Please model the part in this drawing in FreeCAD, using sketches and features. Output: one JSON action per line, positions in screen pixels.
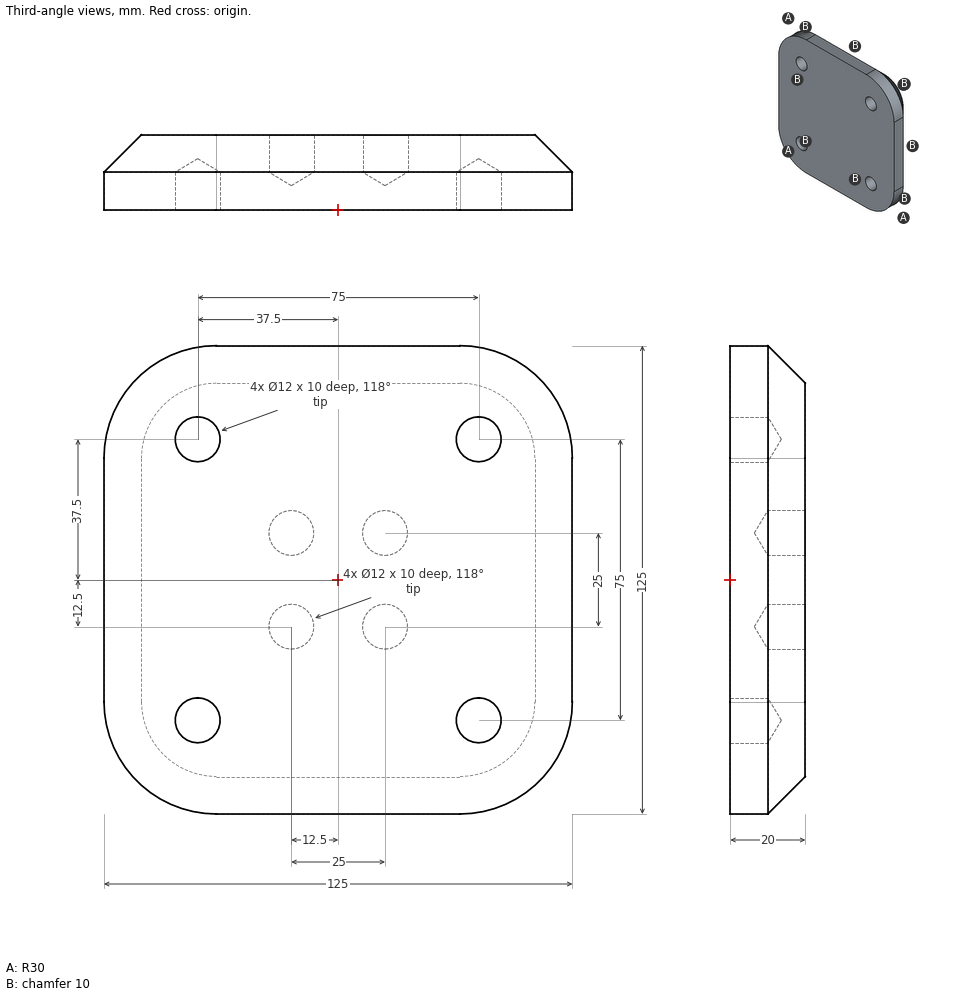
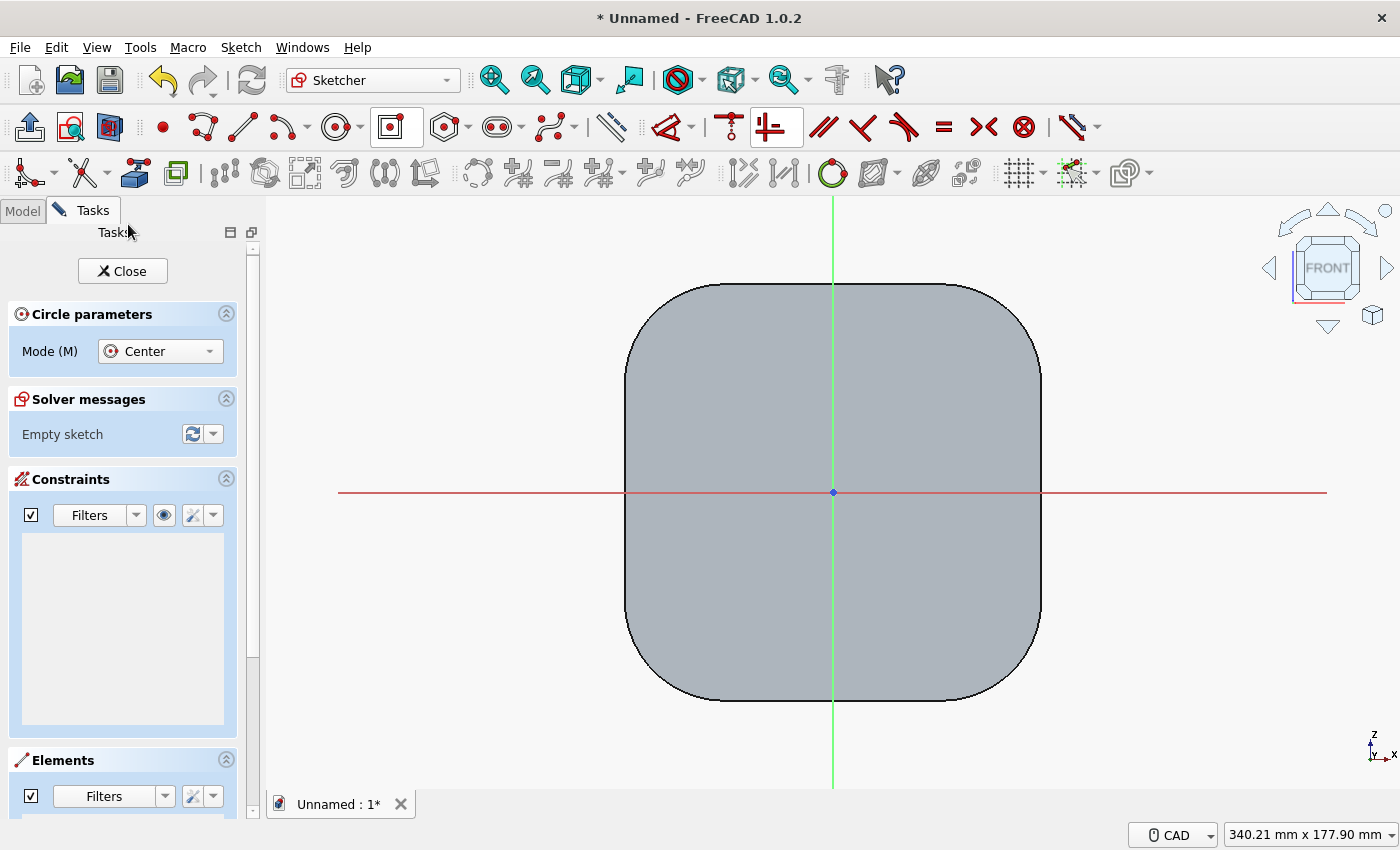
{"action": "left_click", "coordinate": [708, 368]}
{"action": "left_click", "coordinate": [722, 353]}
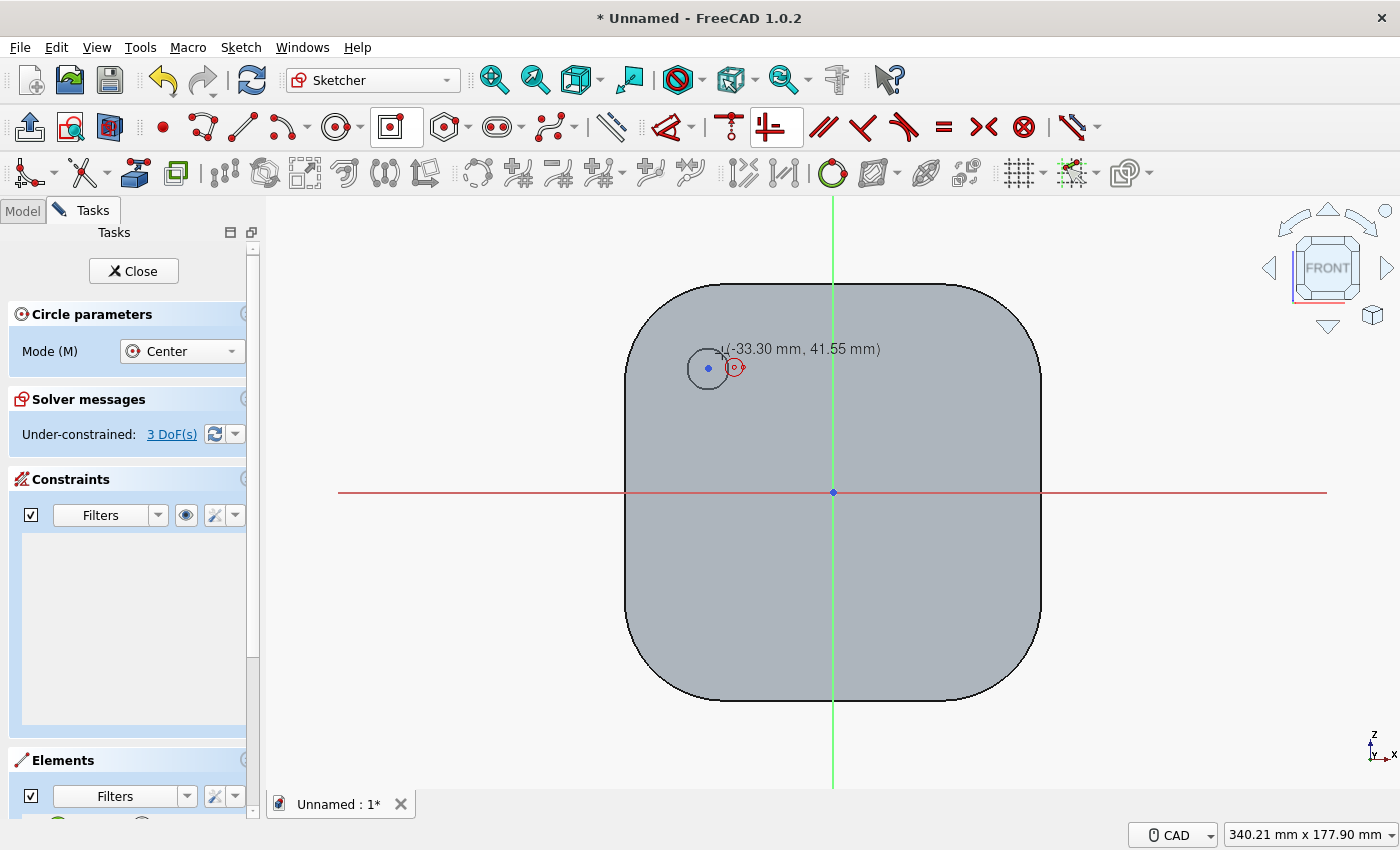
{"action": "left_click", "coordinate": [958, 368]}
{"action": "left_click", "coordinate": [972, 353]}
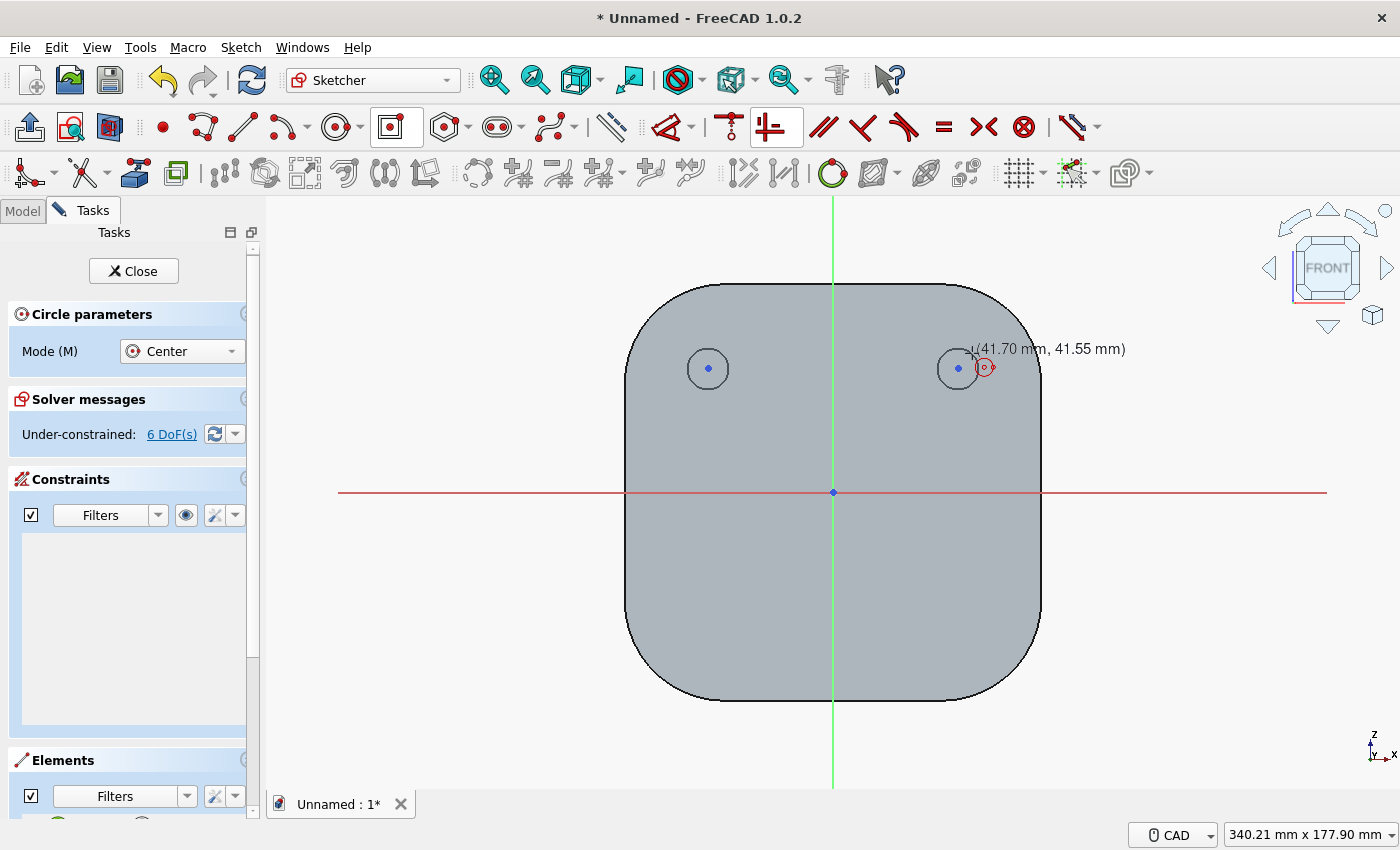
{"action": "left_click", "coordinate": [958, 617]}
{"action": "left_click", "coordinate": [972, 603]}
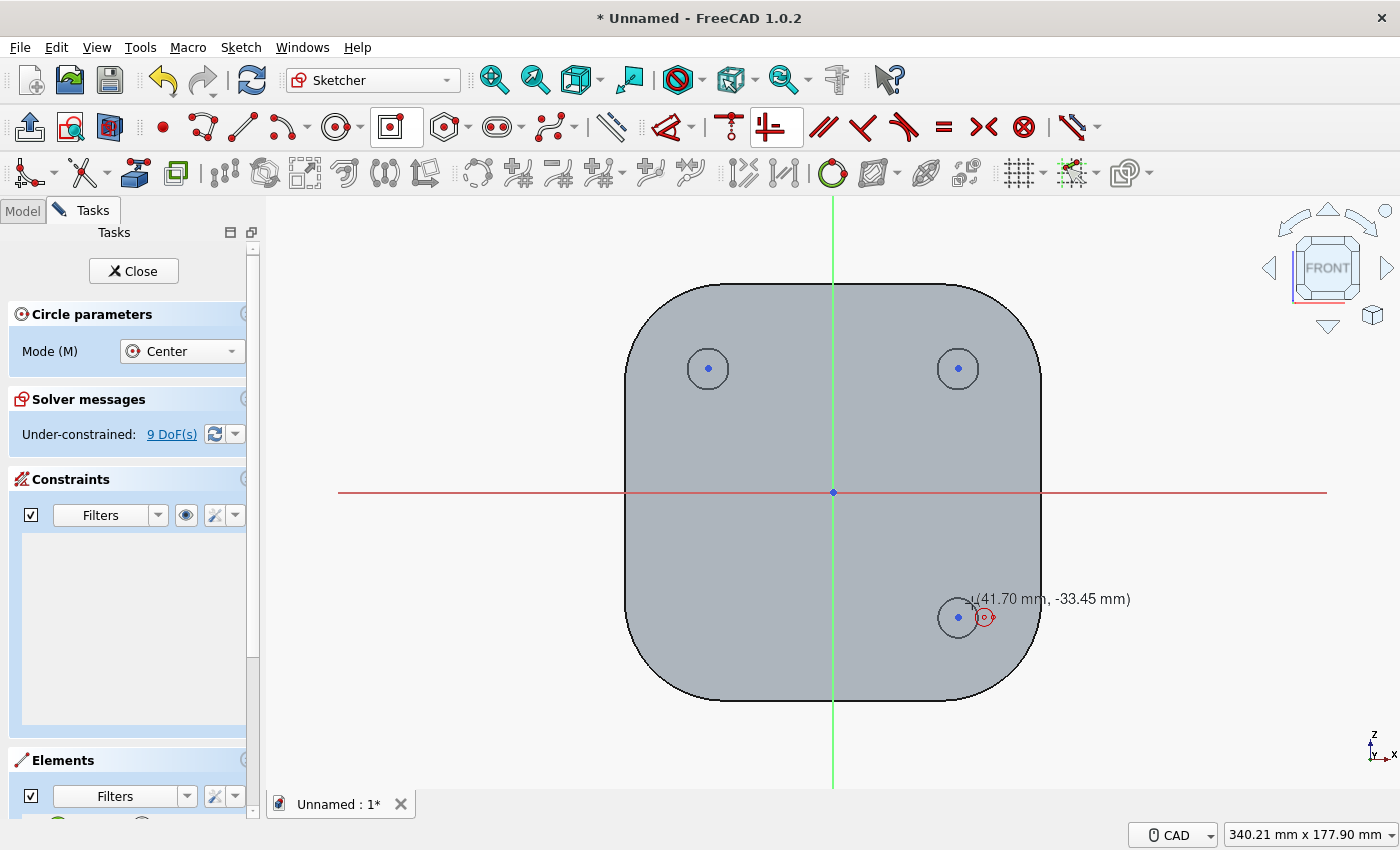
{"action": "left_click", "coordinate": [708, 617]}
{"action": "left_click", "coordinate": [722, 603]}
{"action": "key", "text": "Escape"}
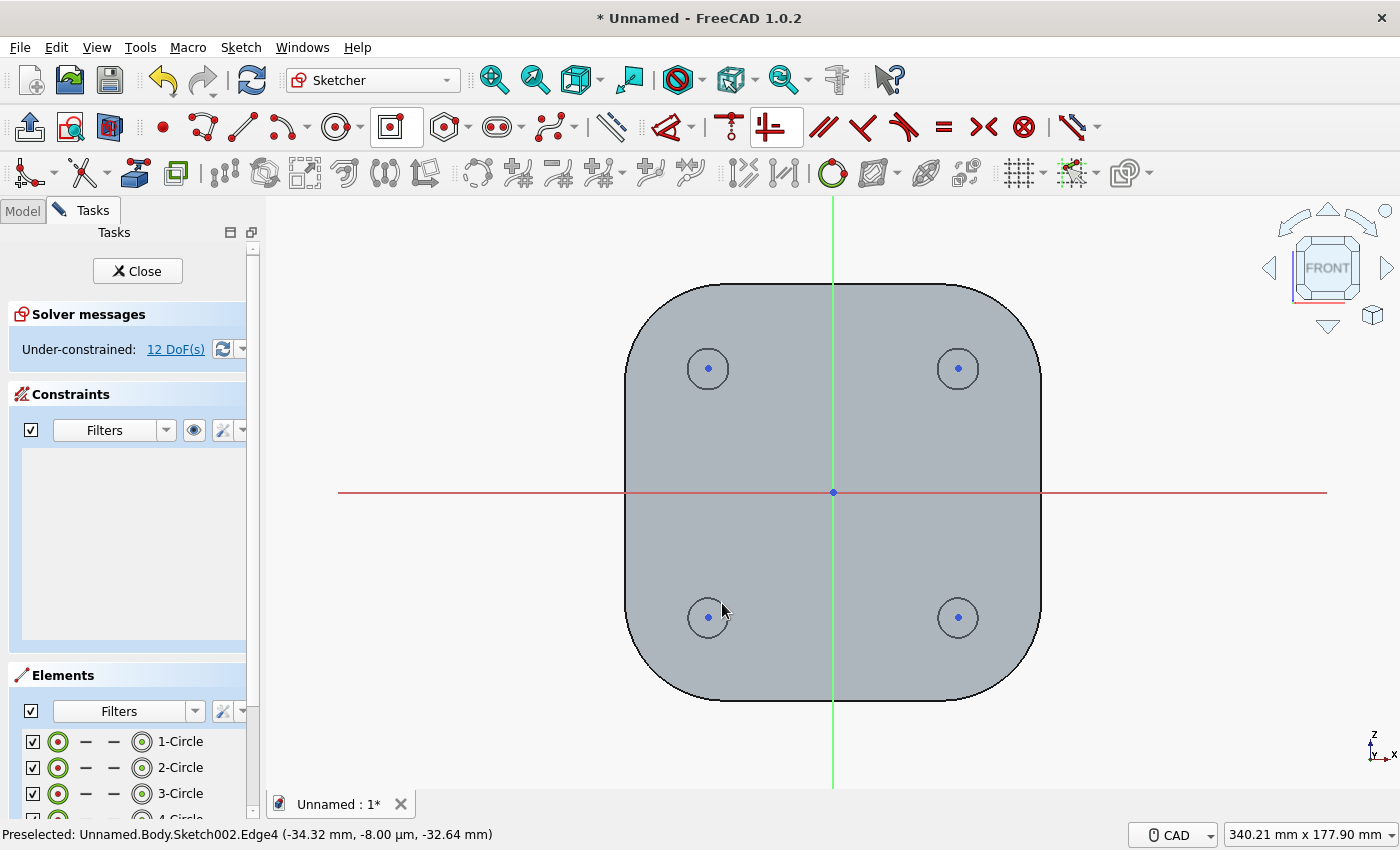
{"action": "left_click", "coordinate": [722, 354]}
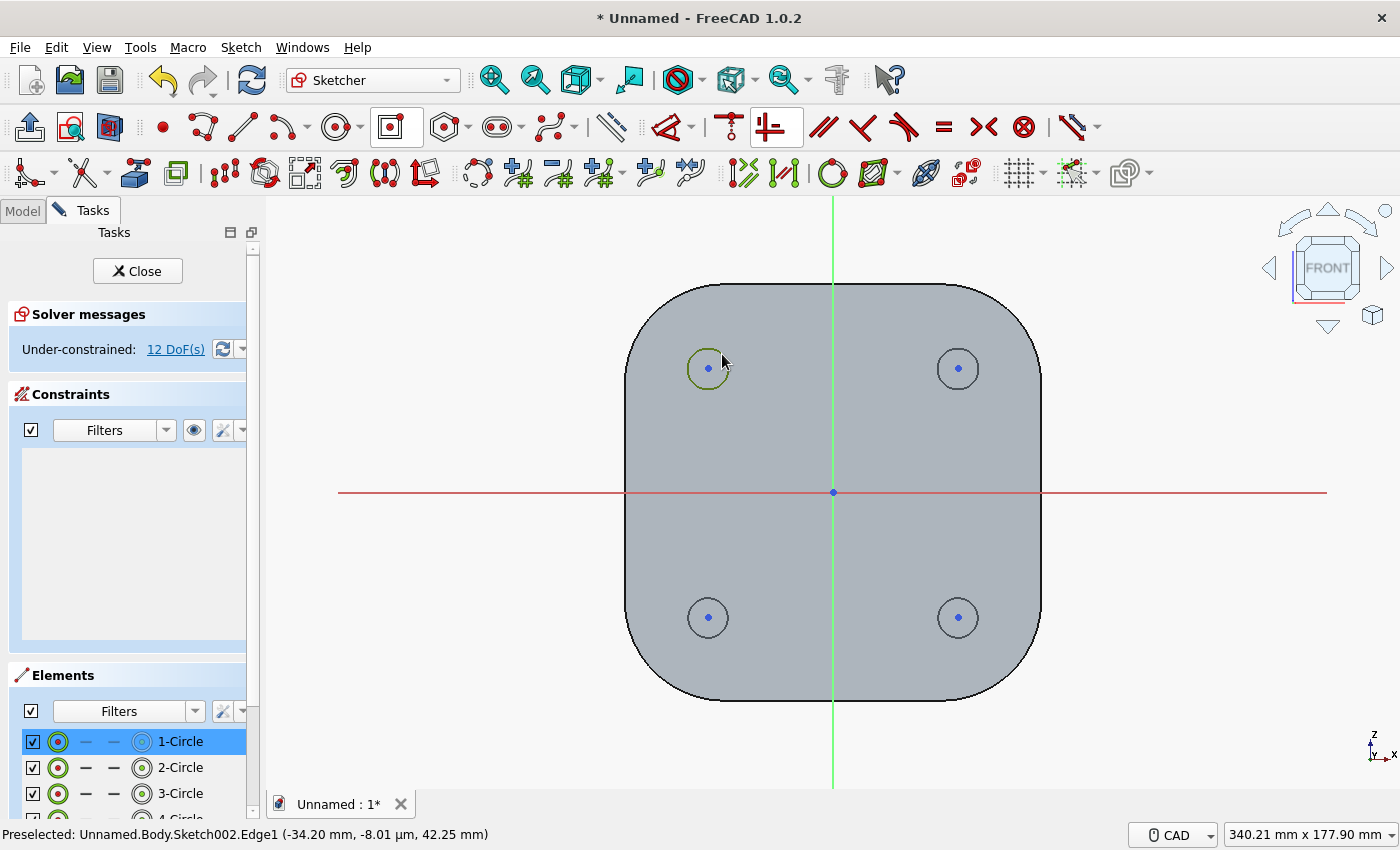
{"action": "left_click", "coordinate": [972, 354]}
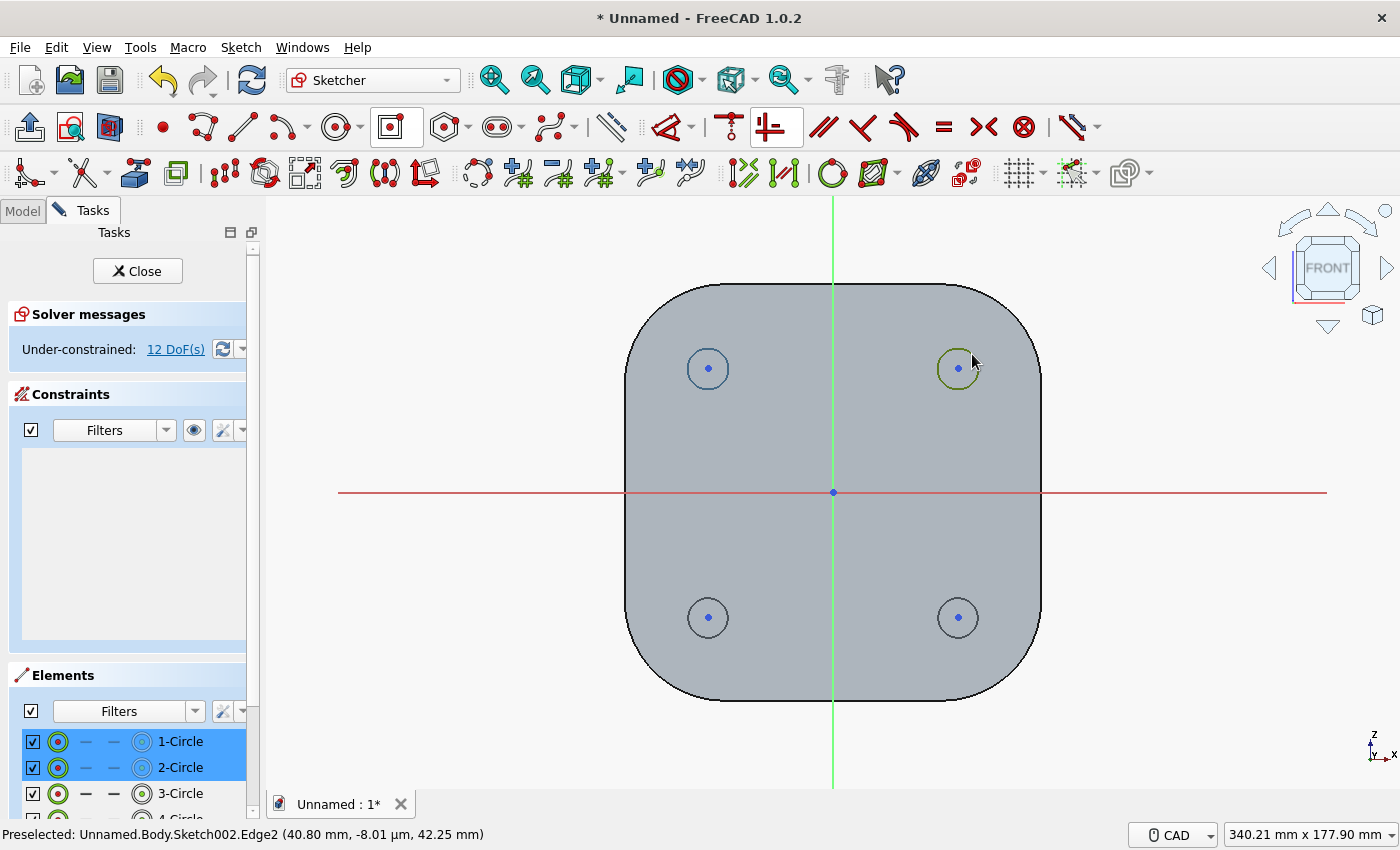
{"action": "left_click", "coordinate": [972, 604]}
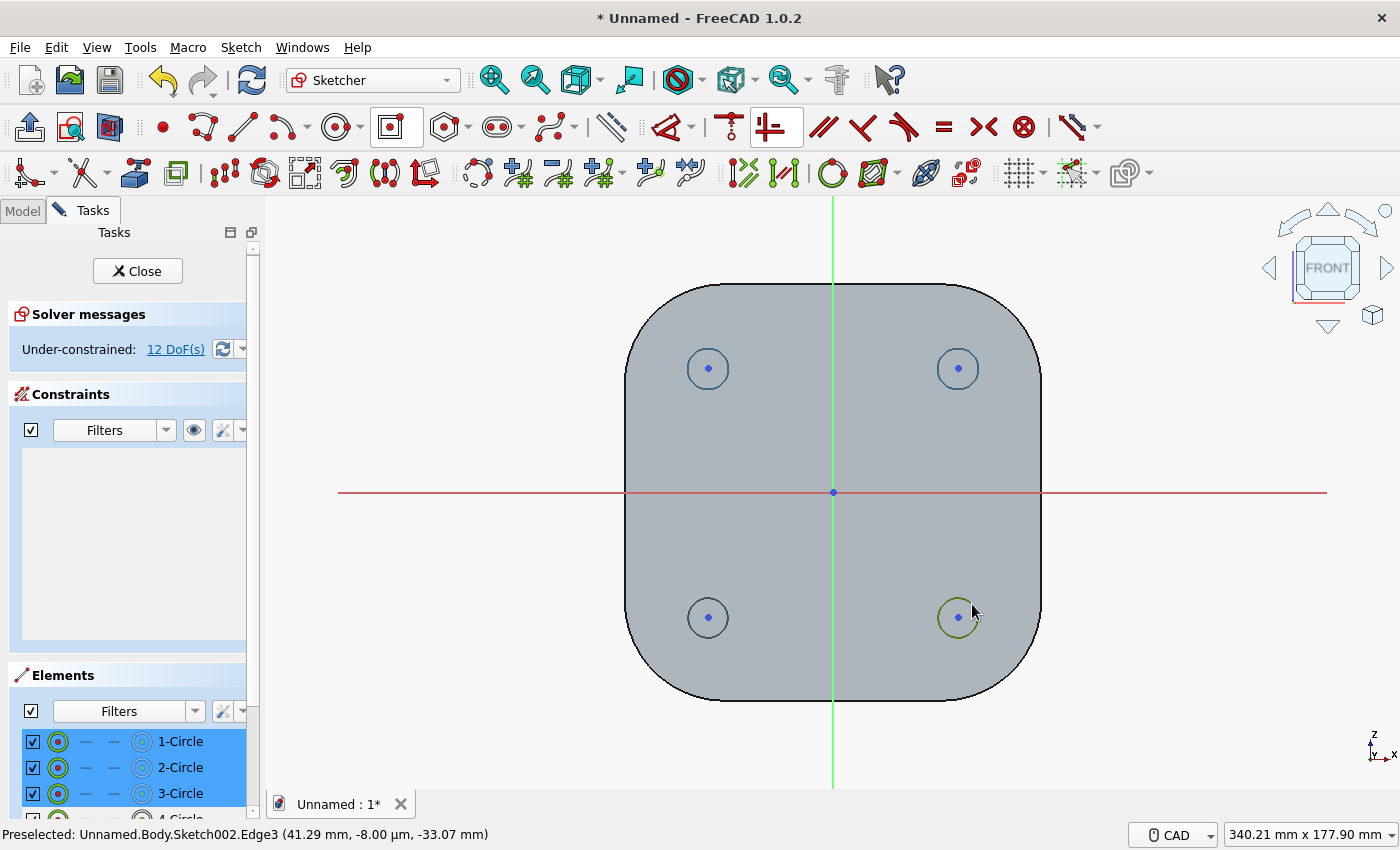
{"action": "left_click", "coordinate": [722, 604]}